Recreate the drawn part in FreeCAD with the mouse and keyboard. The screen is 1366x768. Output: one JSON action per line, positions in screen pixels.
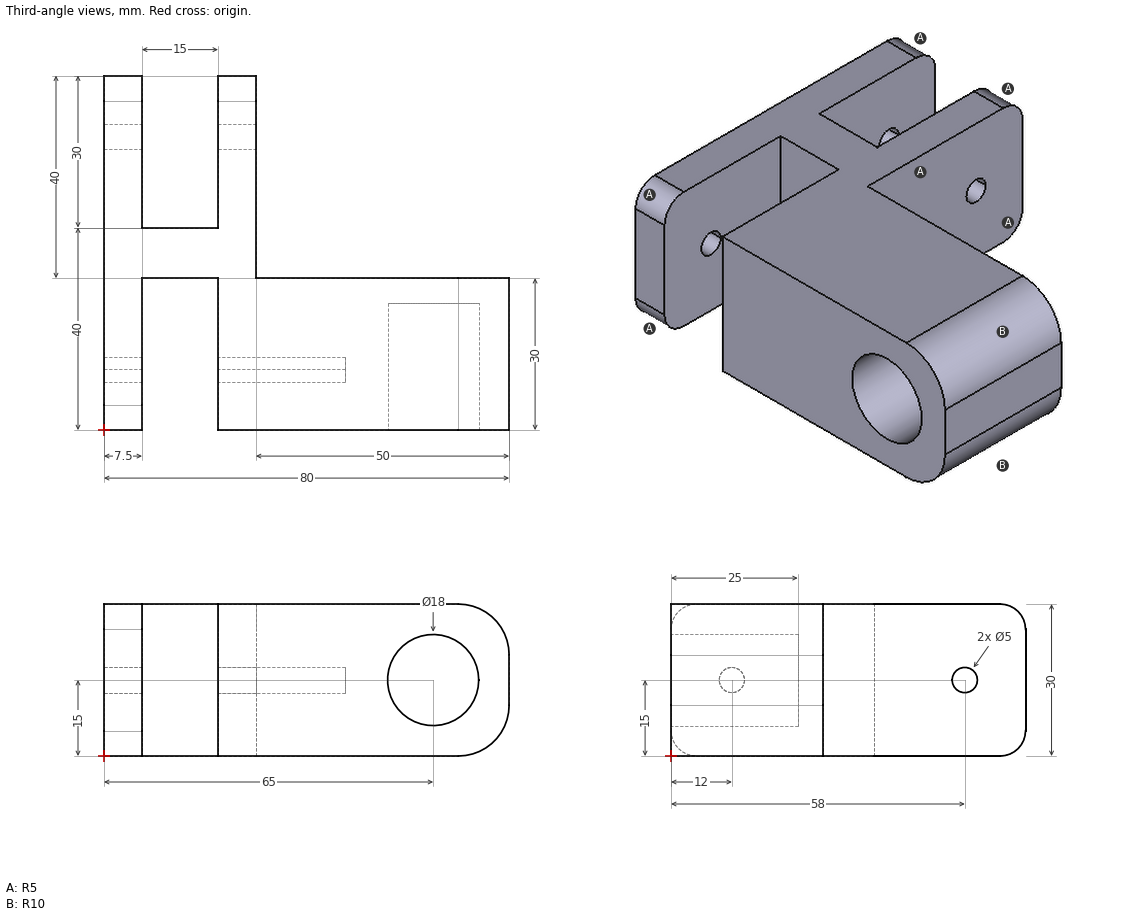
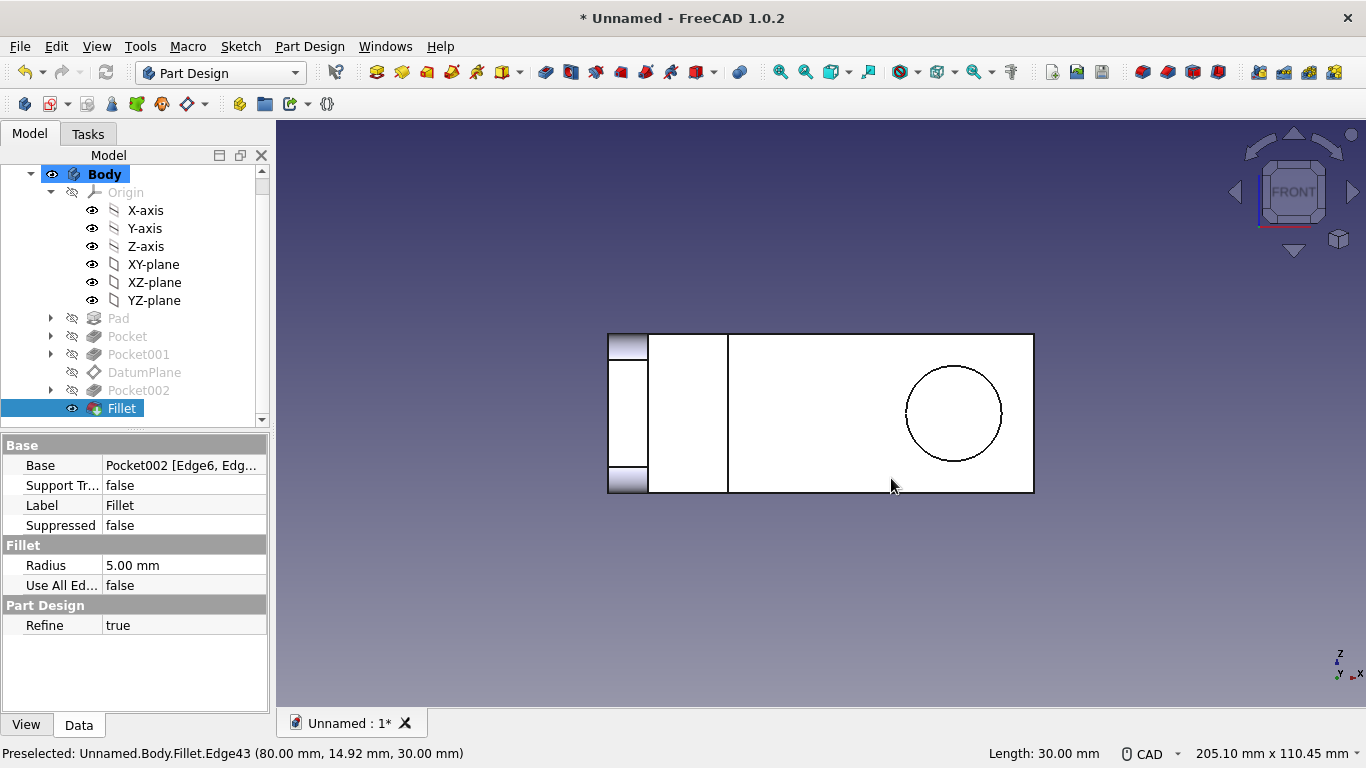
{"action": "left_click", "coordinate": [781, 72]}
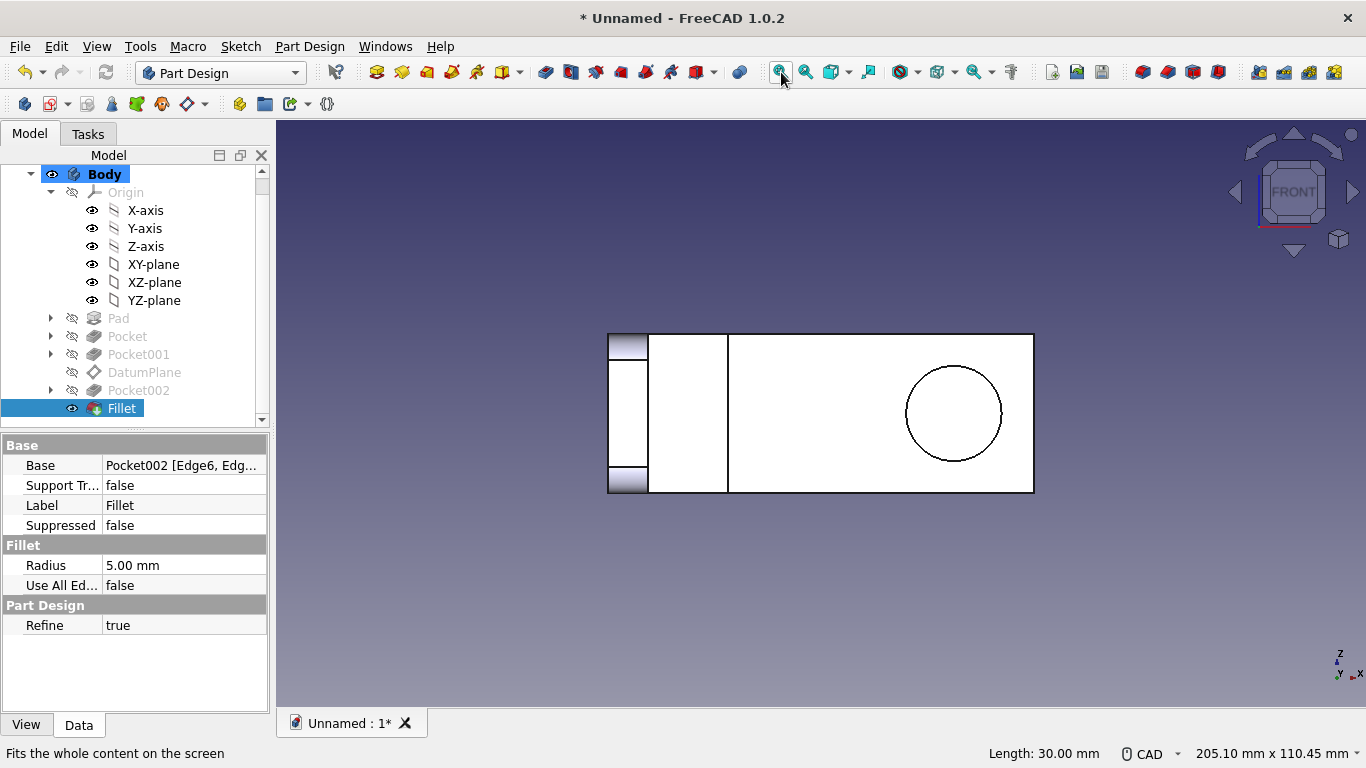
{"action": "key", "text": "3"}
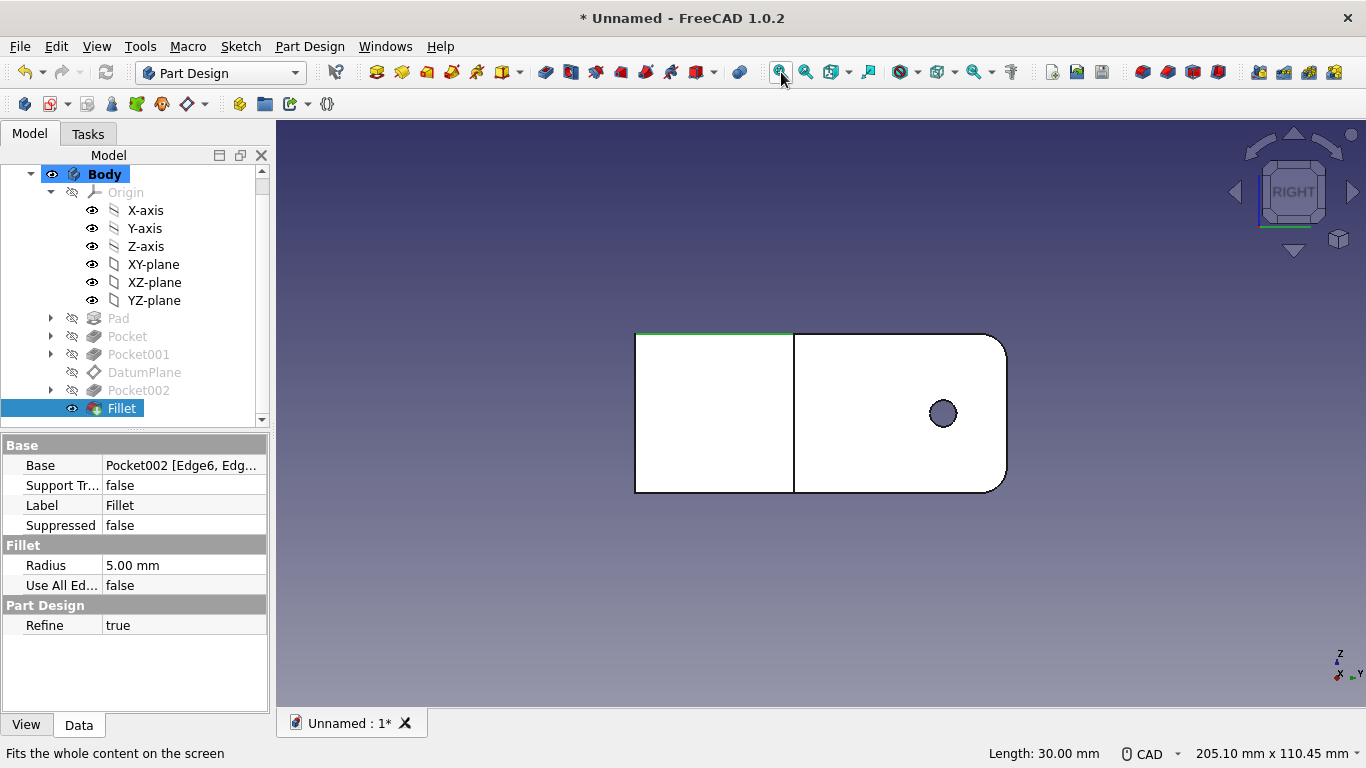
{"action": "key", "text": "v f"}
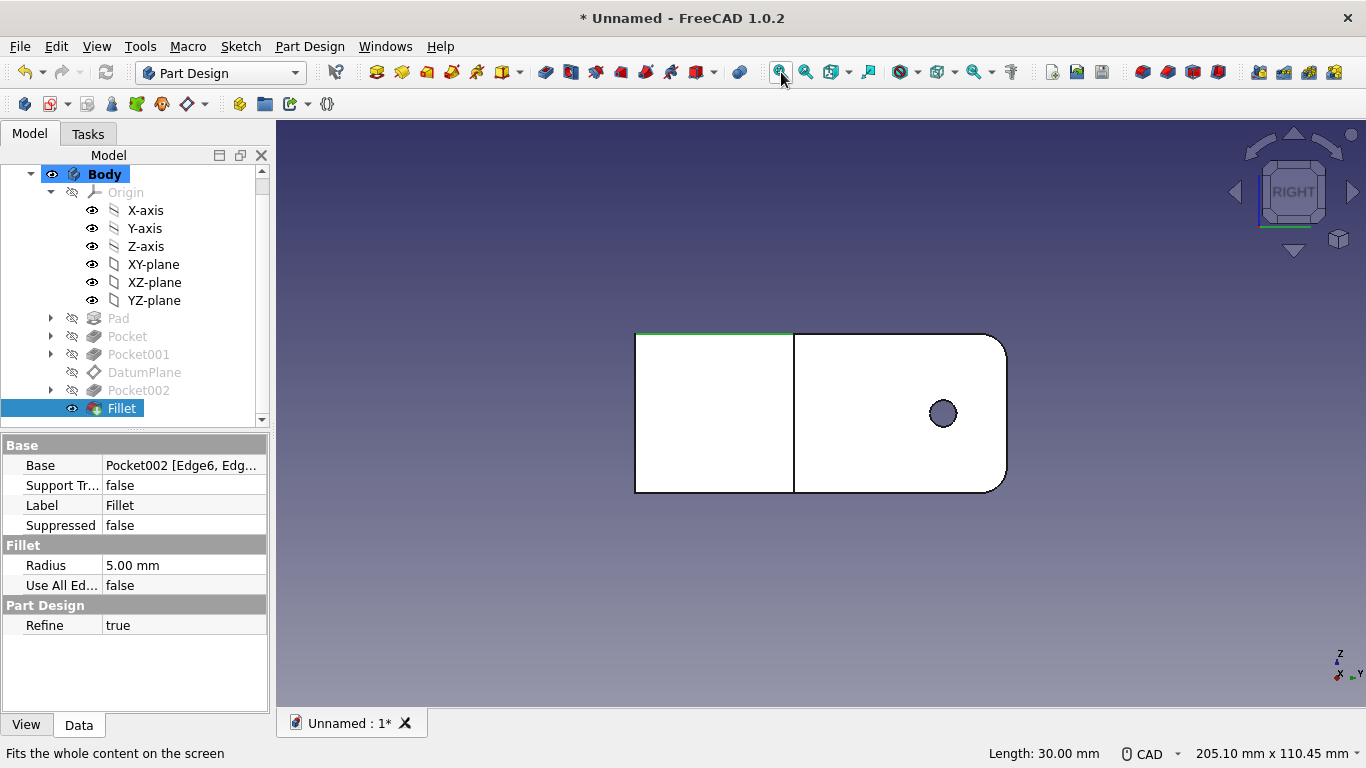
{"action": "left_click", "coordinate": [715, 492], "text": "ctrl"}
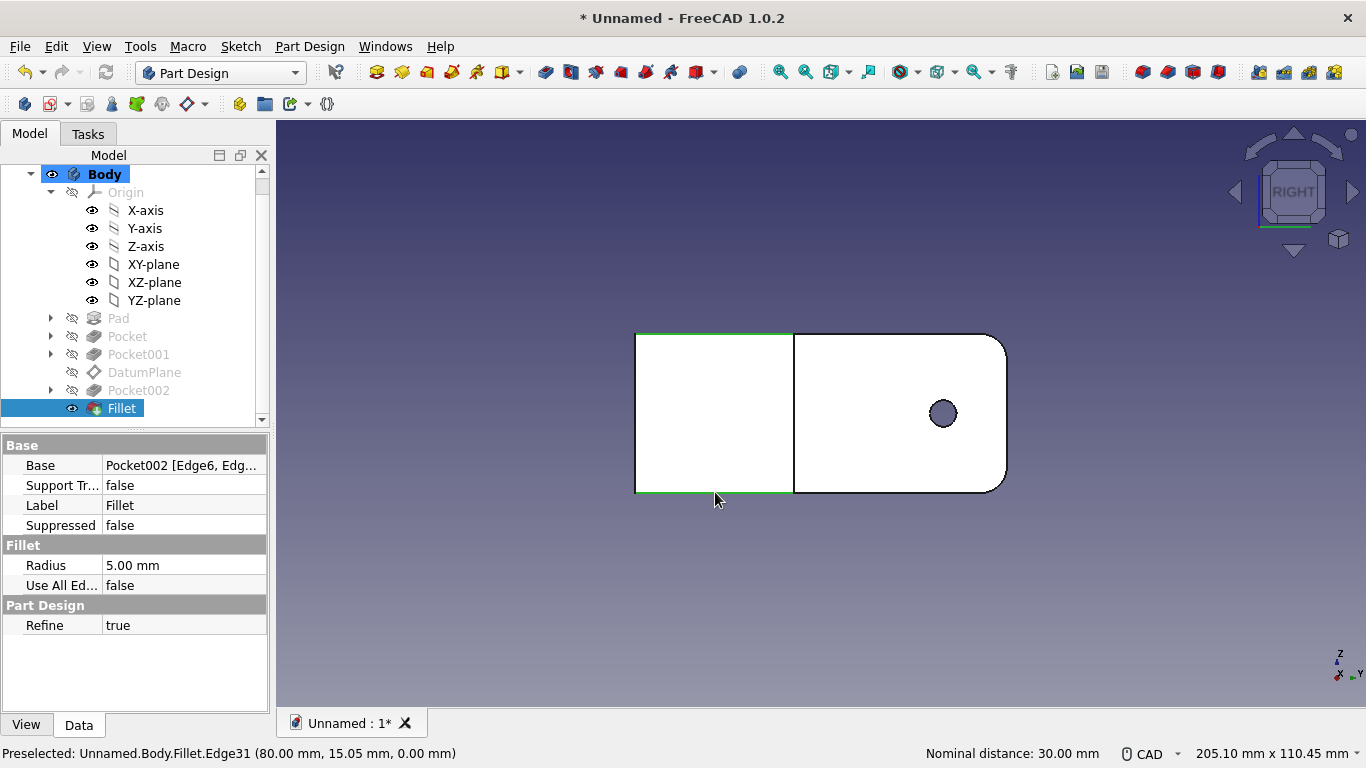
{"action": "left_click", "coordinate": [1143, 72]}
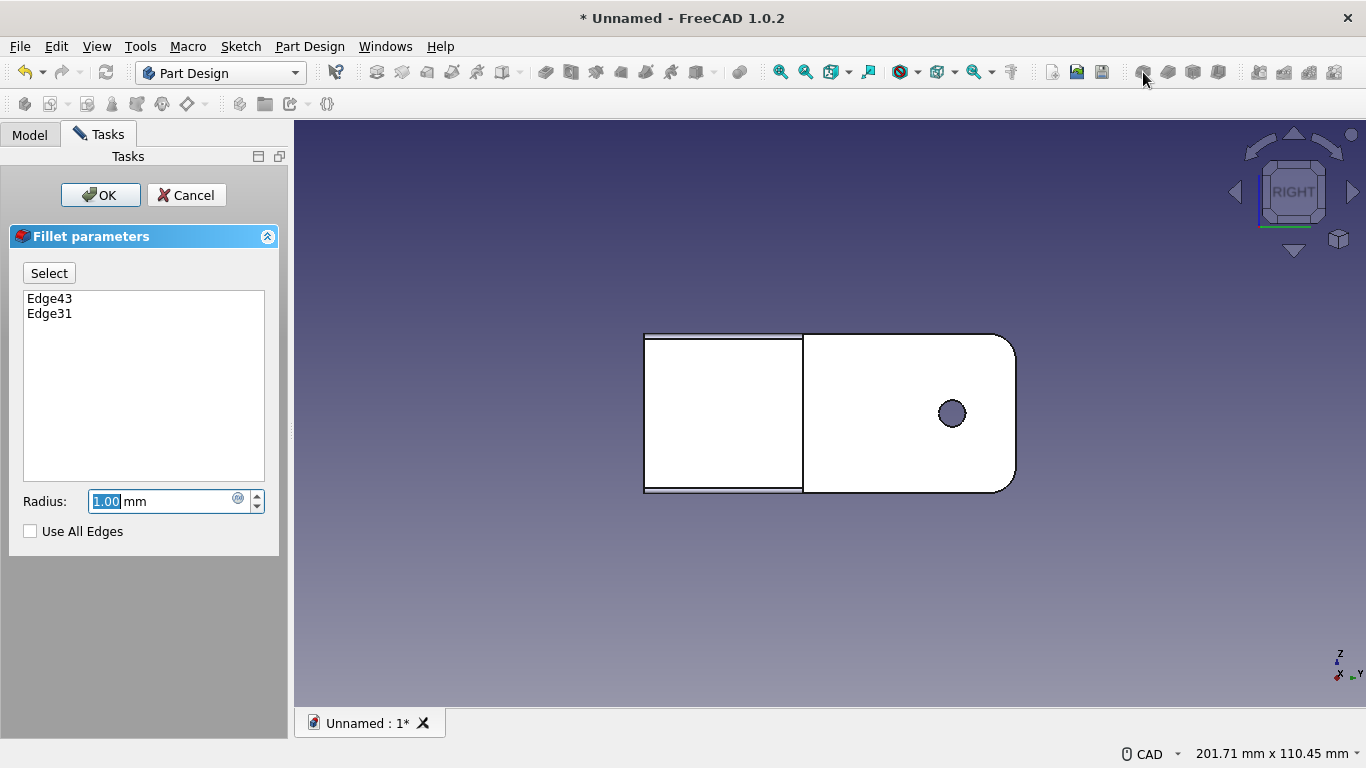
{"action": "type", "text": "10"}
{"action": "key", "text": "Tab"}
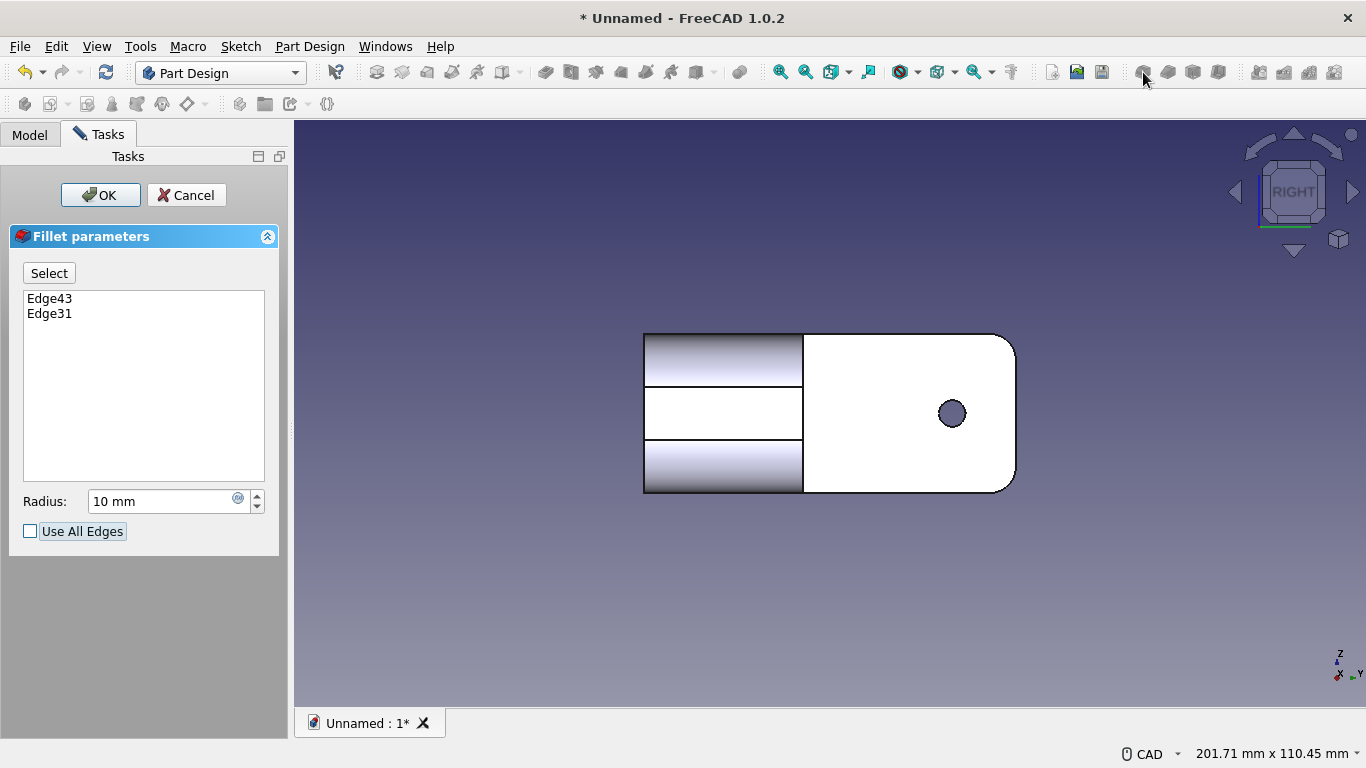
{"action": "left_click", "coordinate": [101, 195]}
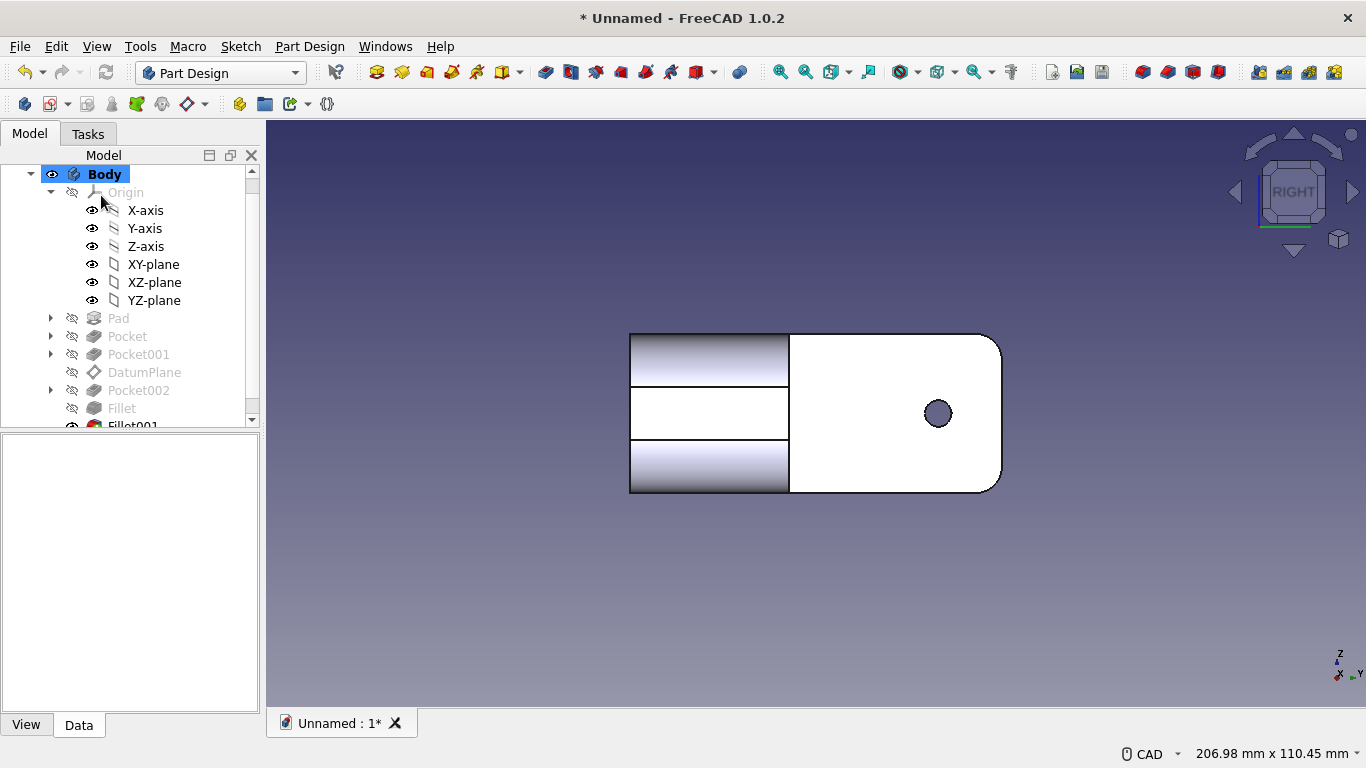
{"action": "key", "text": "0"}